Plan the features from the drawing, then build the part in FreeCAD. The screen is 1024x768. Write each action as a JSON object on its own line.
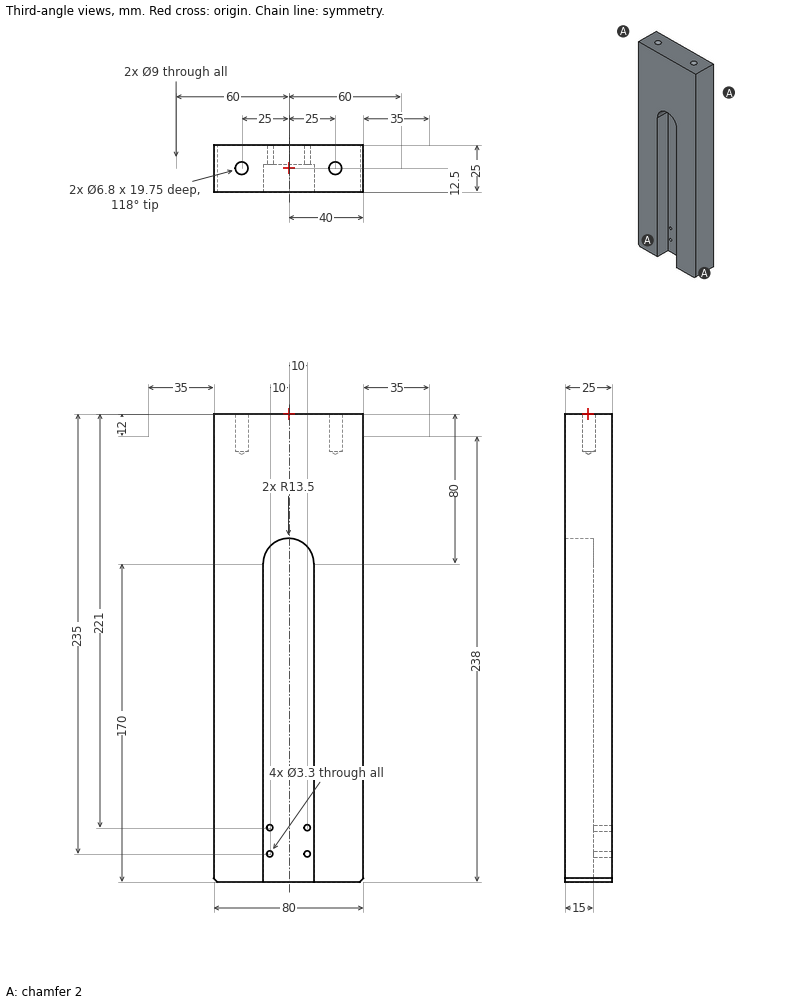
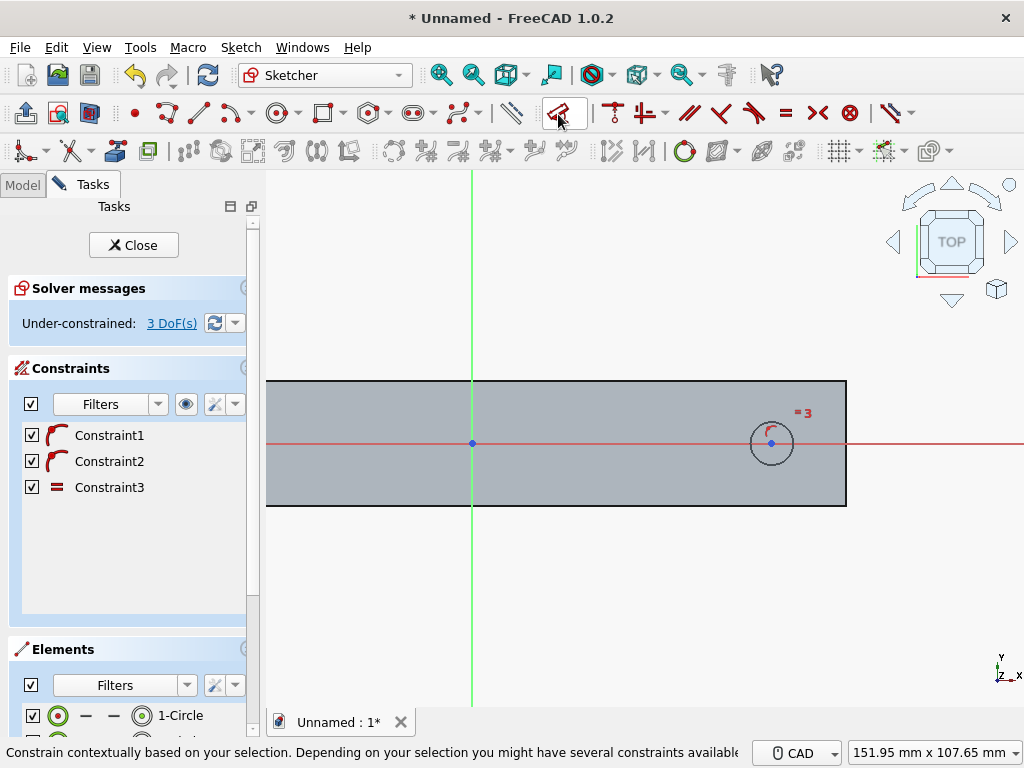
{"action": "scroll", "coordinate": [788, 428], "scroll_direction": "down", "scroll_amount": 2}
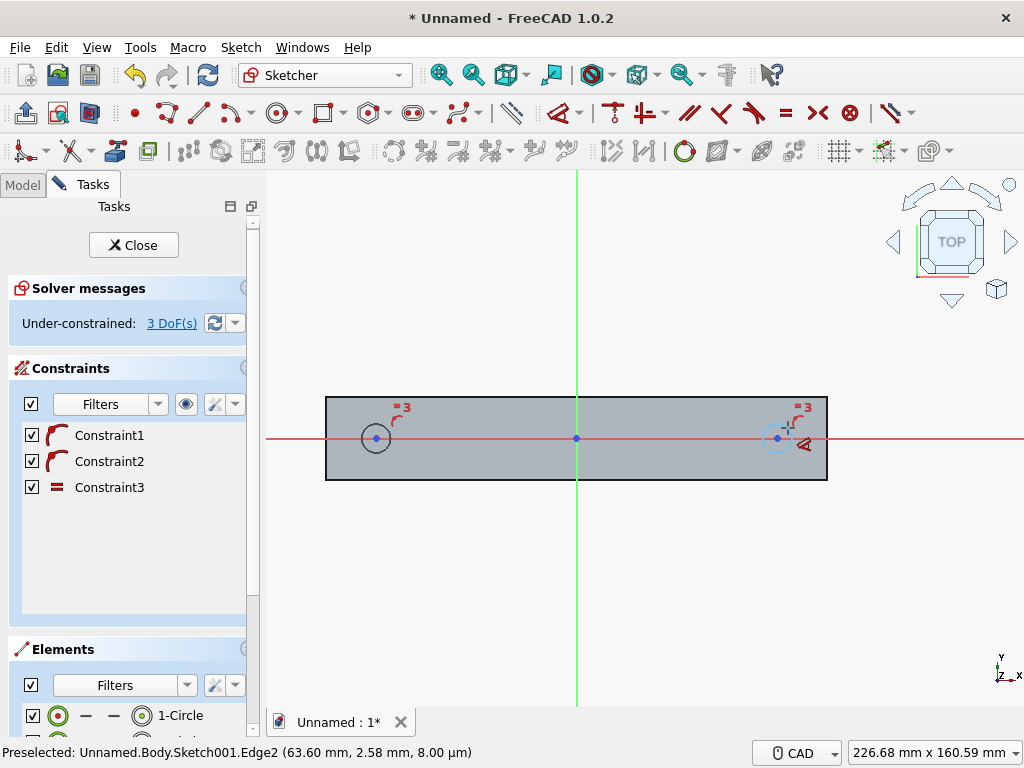
{"action": "scroll", "coordinate": [386, 428], "scroll_direction": "up", "scroll_amount": 2}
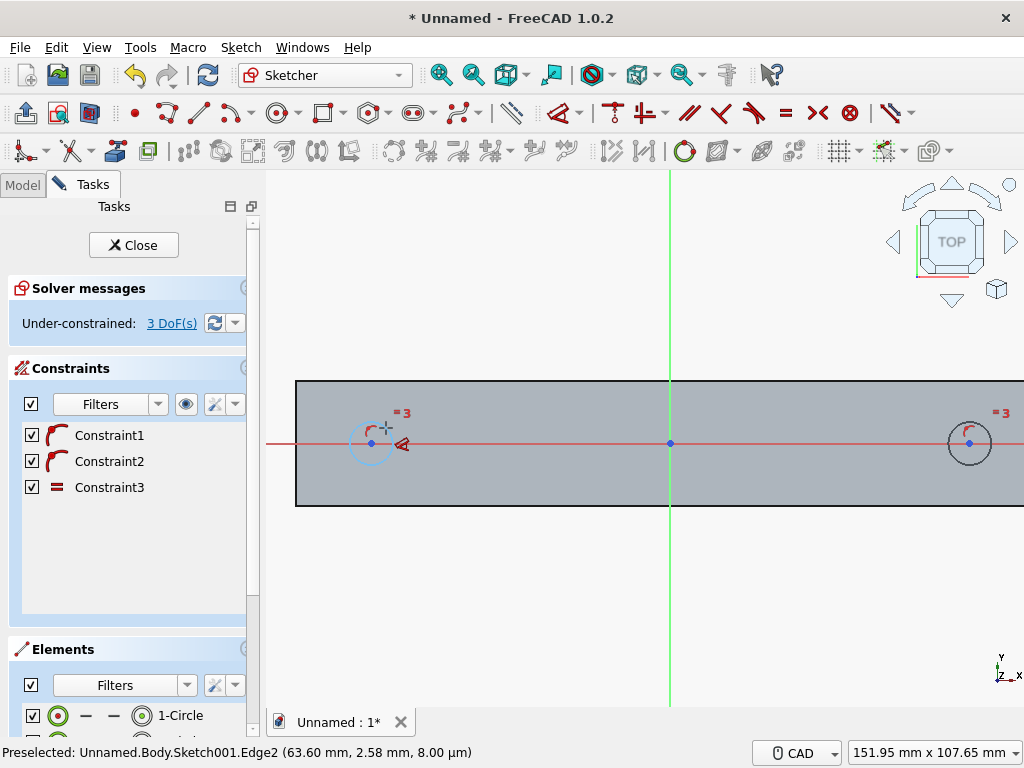
{"action": "left_click", "coordinate": [386, 428]}
{"action": "left_click", "coordinate": [408, 405]}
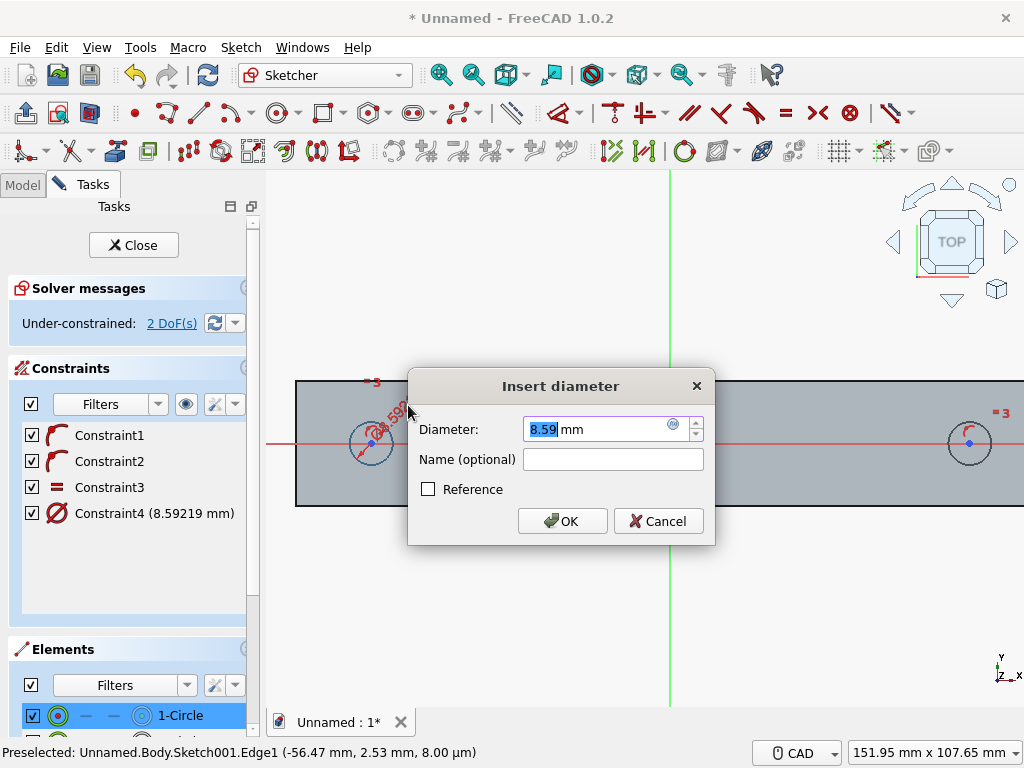
{"action": "type", "text": "9"}
{"action": "key", "text": "Return"}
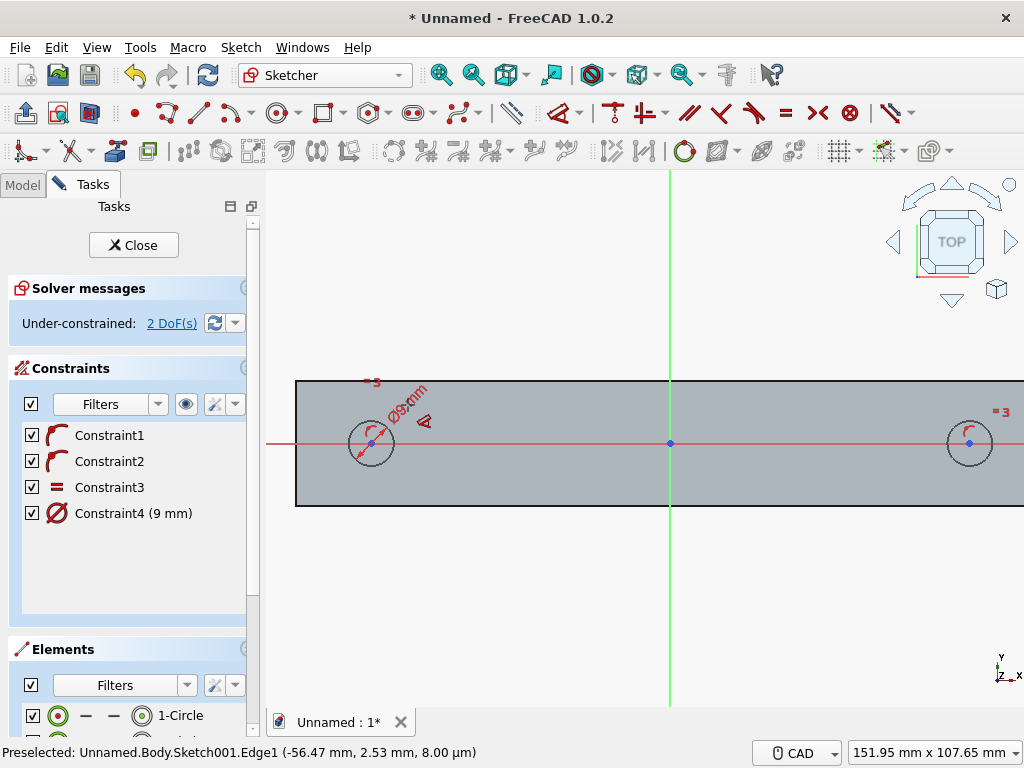
{"action": "left_click", "coordinate": [371, 444]}
{"action": "left_click", "coordinate": [521, 478]}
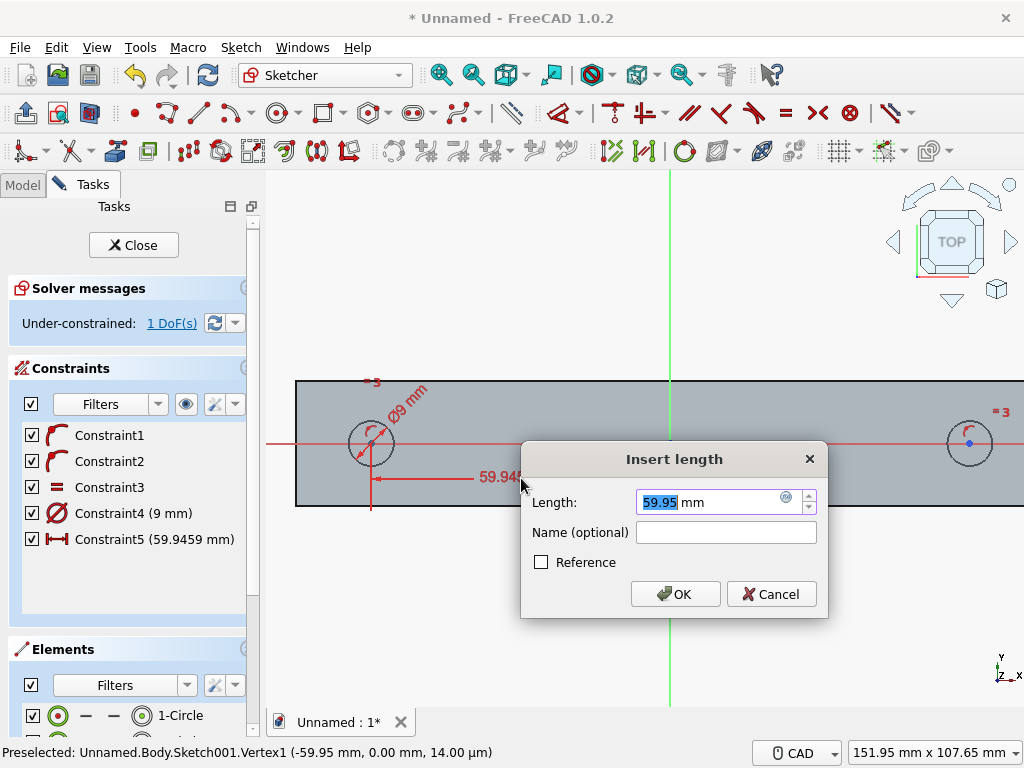
{"action": "type", "text": "60"}
{"action": "key", "text": "Return"}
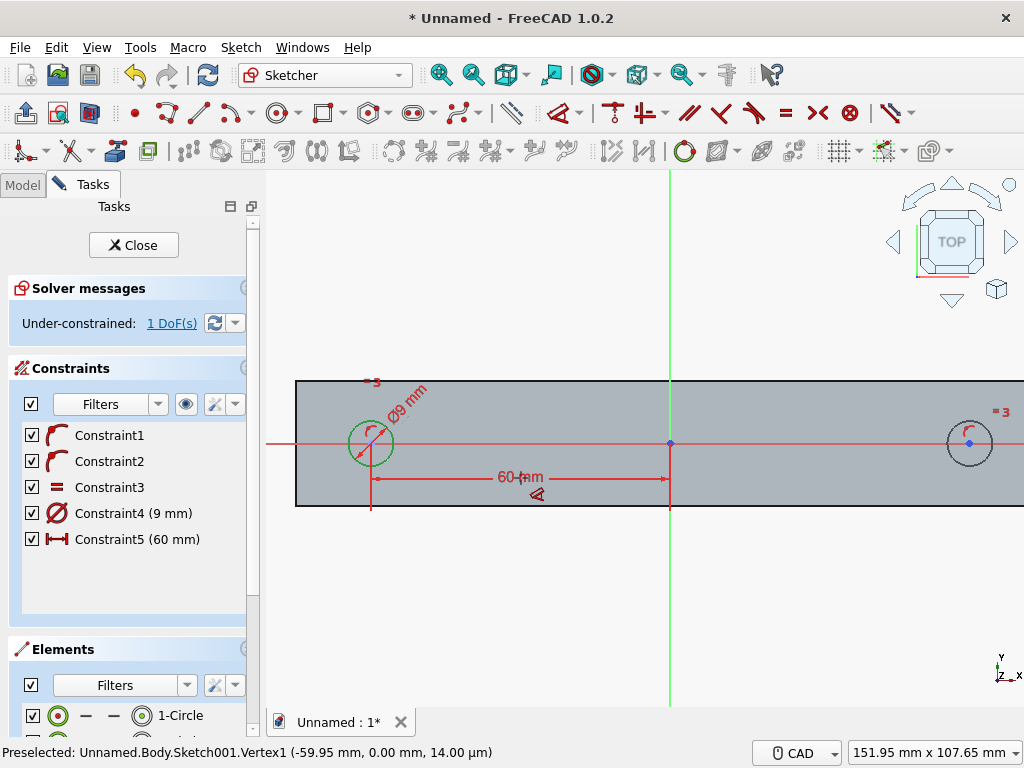
{"action": "scroll", "coordinate": [386, 428], "scroll_direction": "down", "scroll_amount": 2}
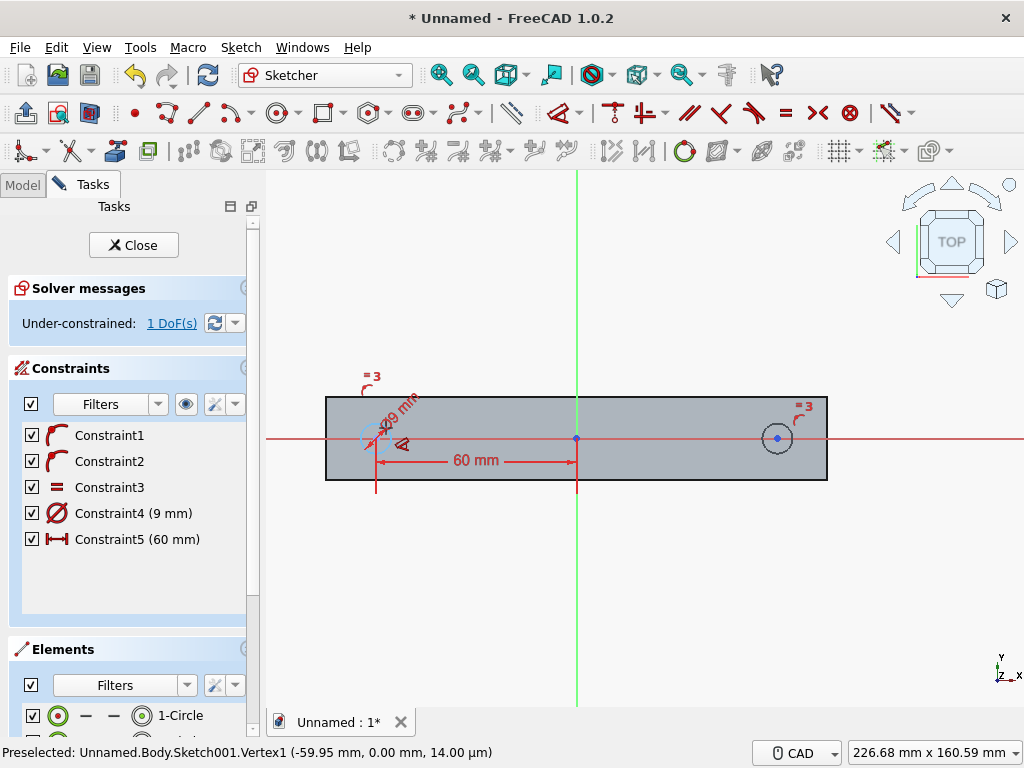
{"action": "left_click", "coordinate": [777, 439]}
{"action": "left_click", "coordinate": [677, 473]}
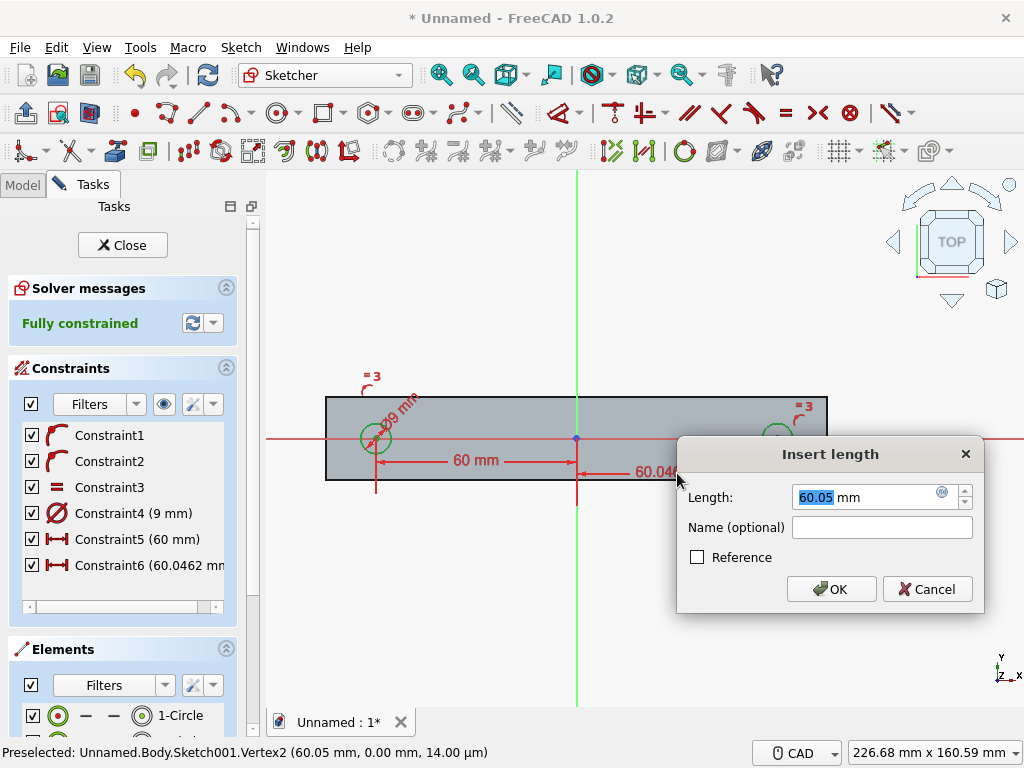
{"action": "type", "text": "60"}
{"action": "key", "text": "Return"}
{"action": "key", "text": "Escape"}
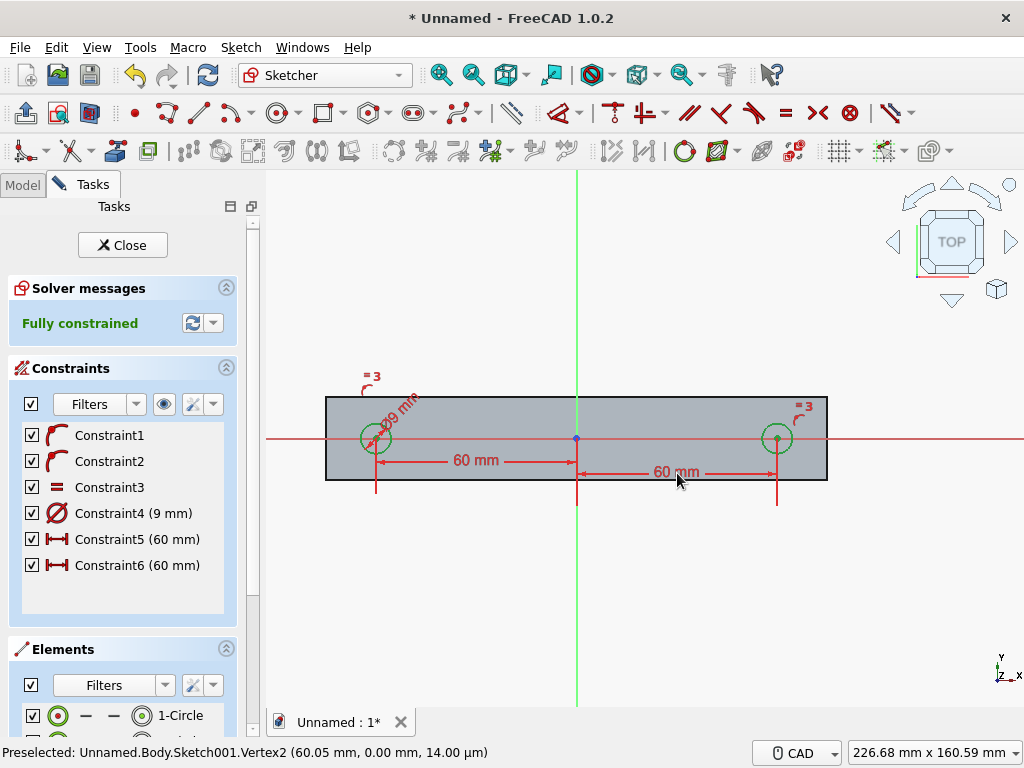
{"action": "left_click", "coordinate": [123, 245]}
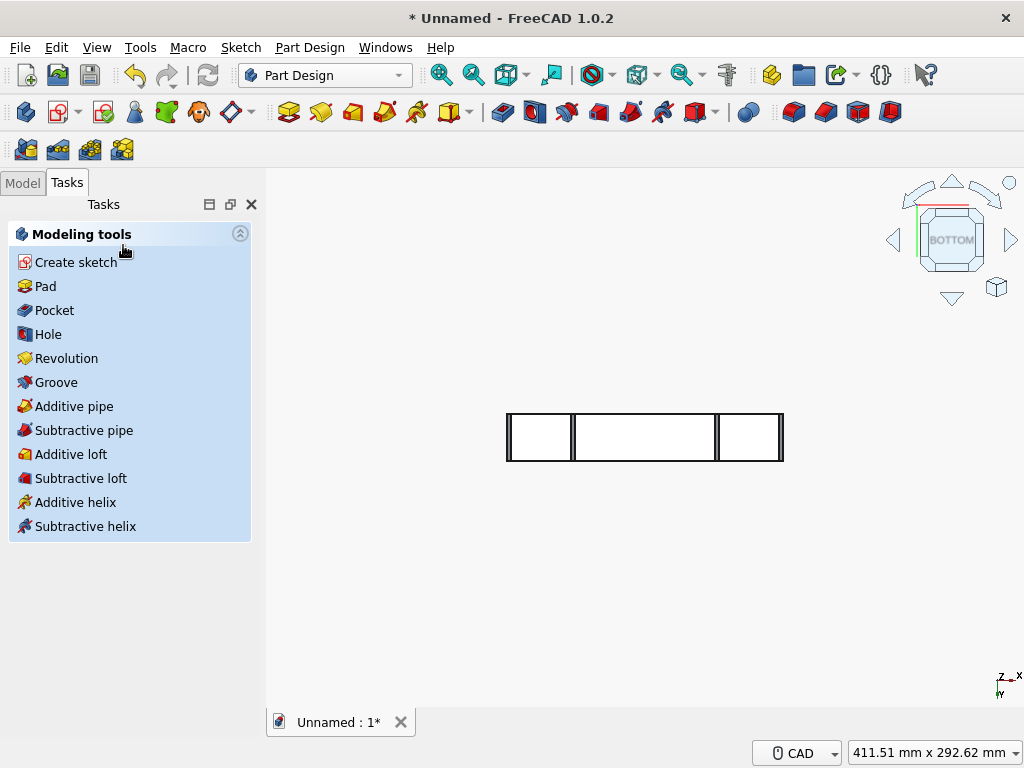
{"action": "left_click", "coordinate": [536, 112]}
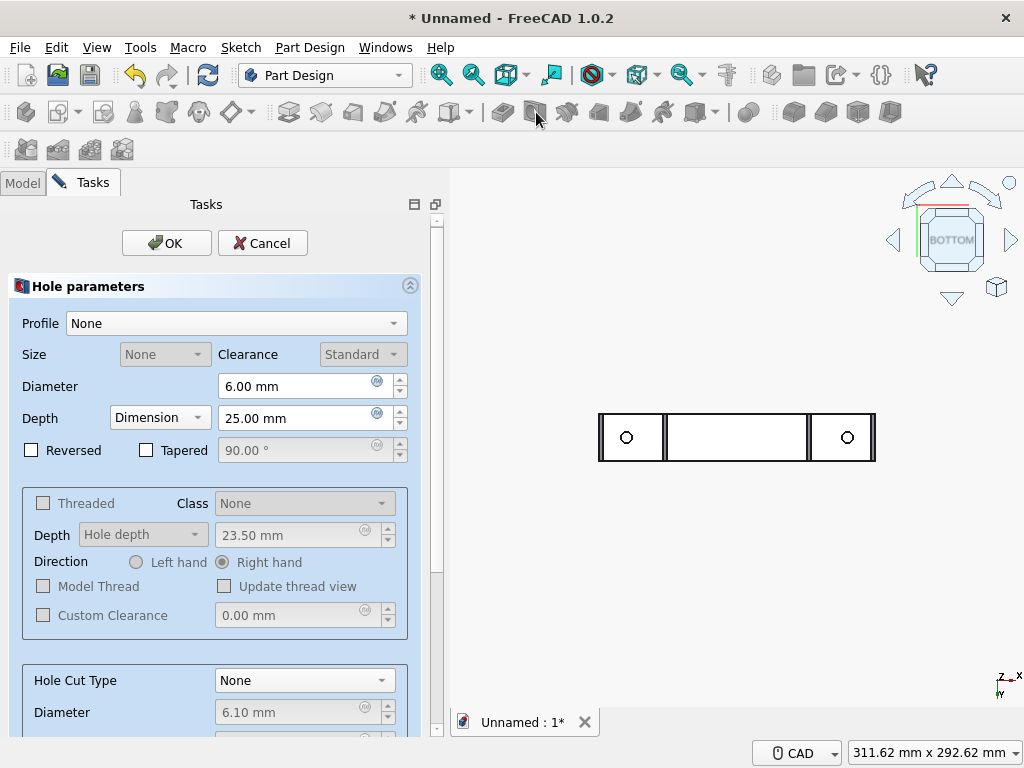
{"action": "triple_click", "coordinate": [305, 386]}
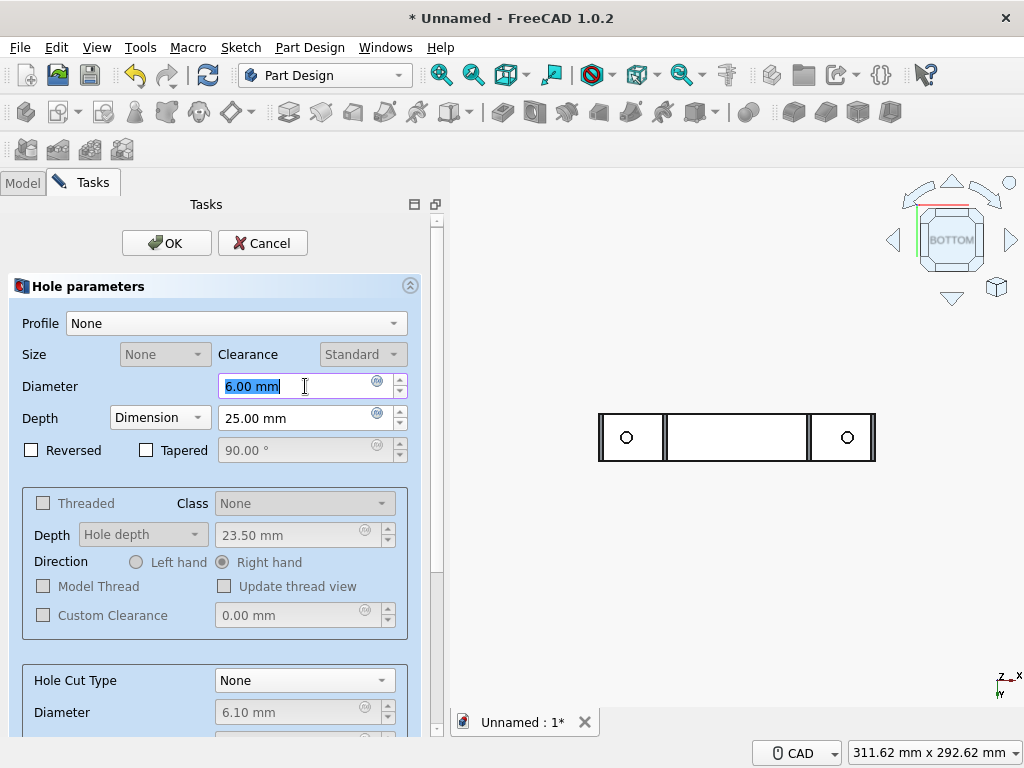
{"action": "type", "text": "9"}
{"action": "key", "text": "Tab"}